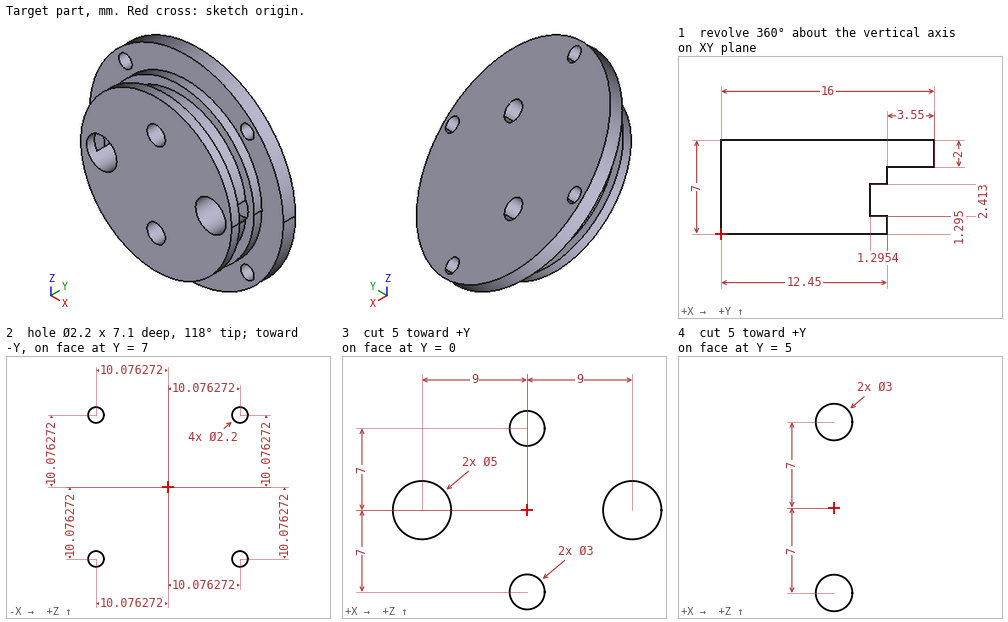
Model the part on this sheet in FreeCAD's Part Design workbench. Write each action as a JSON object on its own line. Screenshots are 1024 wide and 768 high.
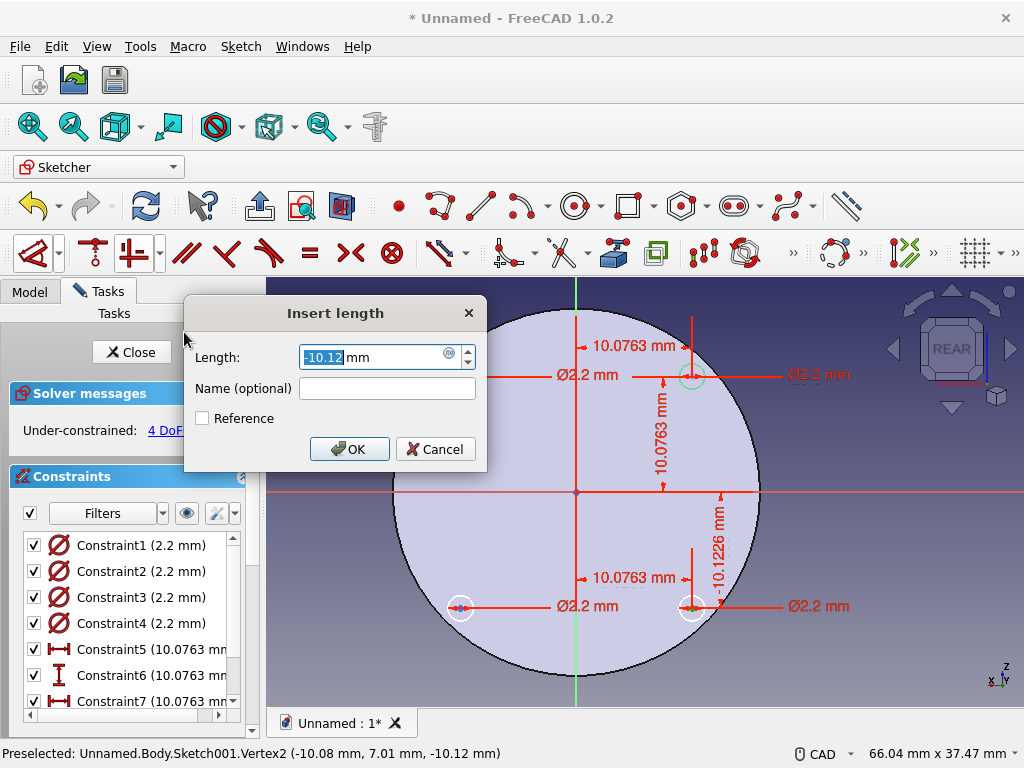
{"action": "type", "text": "-10.076272"}
{"action": "key", "text": "Return"}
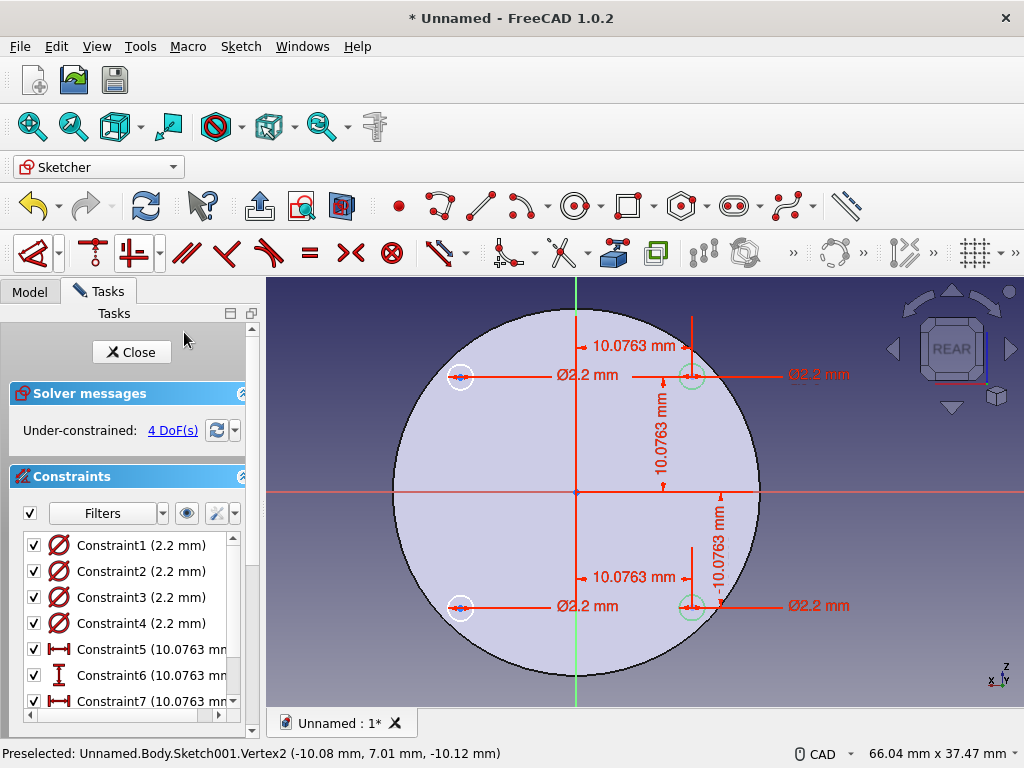
{"action": "left_click", "coordinate": [461, 608]}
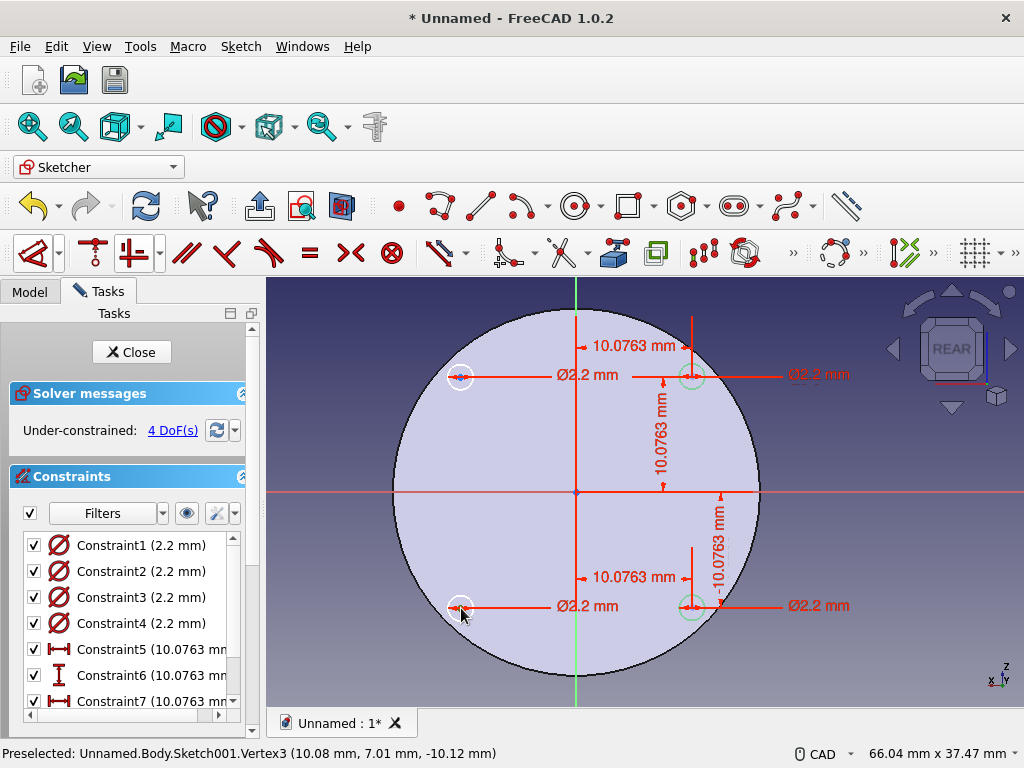
{"action": "left_click", "coordinate": [58, 254]}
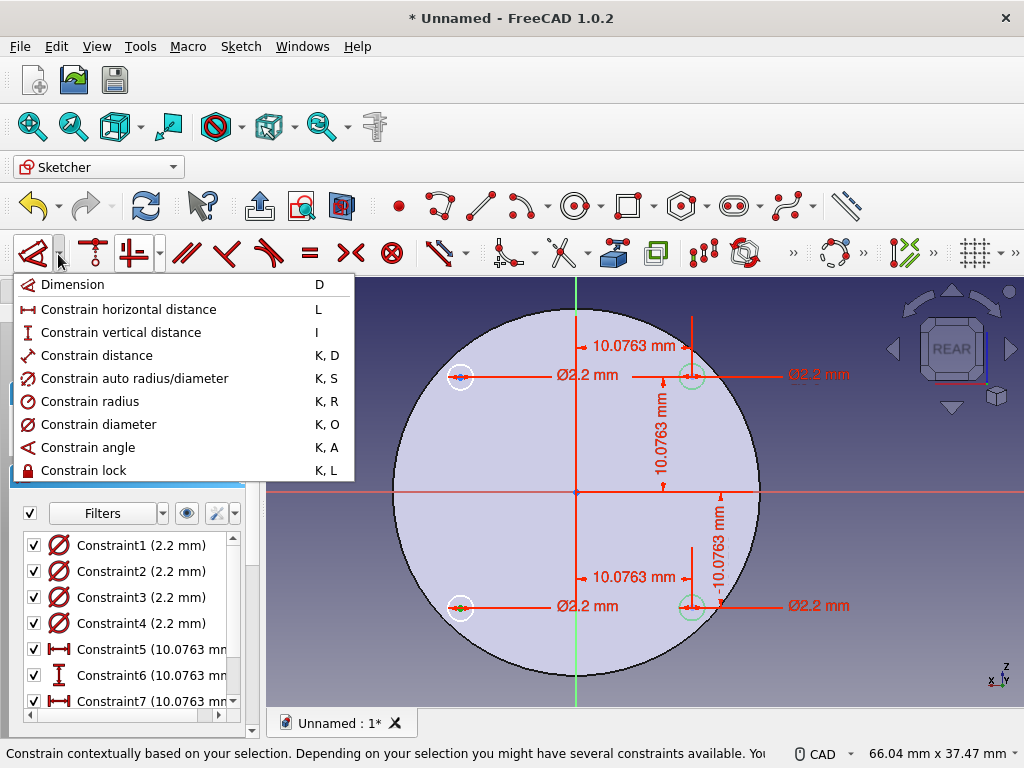
{"action": "left_click", "coordinate": [184, 310]}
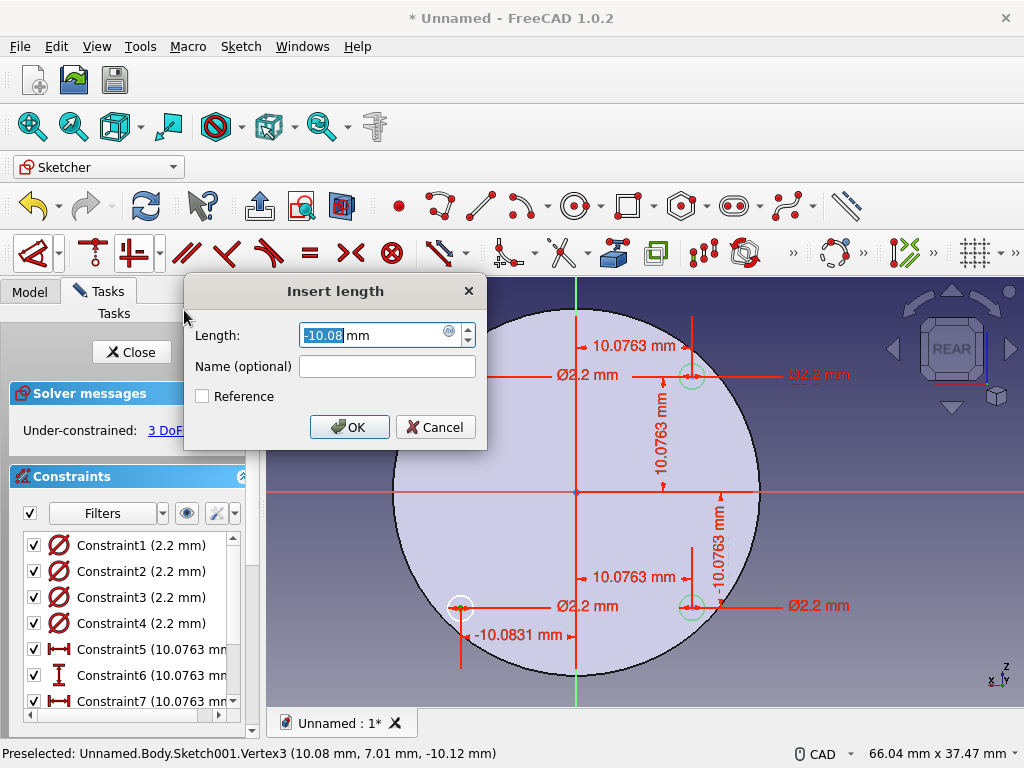
{"action": "type", "text": "-10.076272"}
{"action": "key", "text": "Return"}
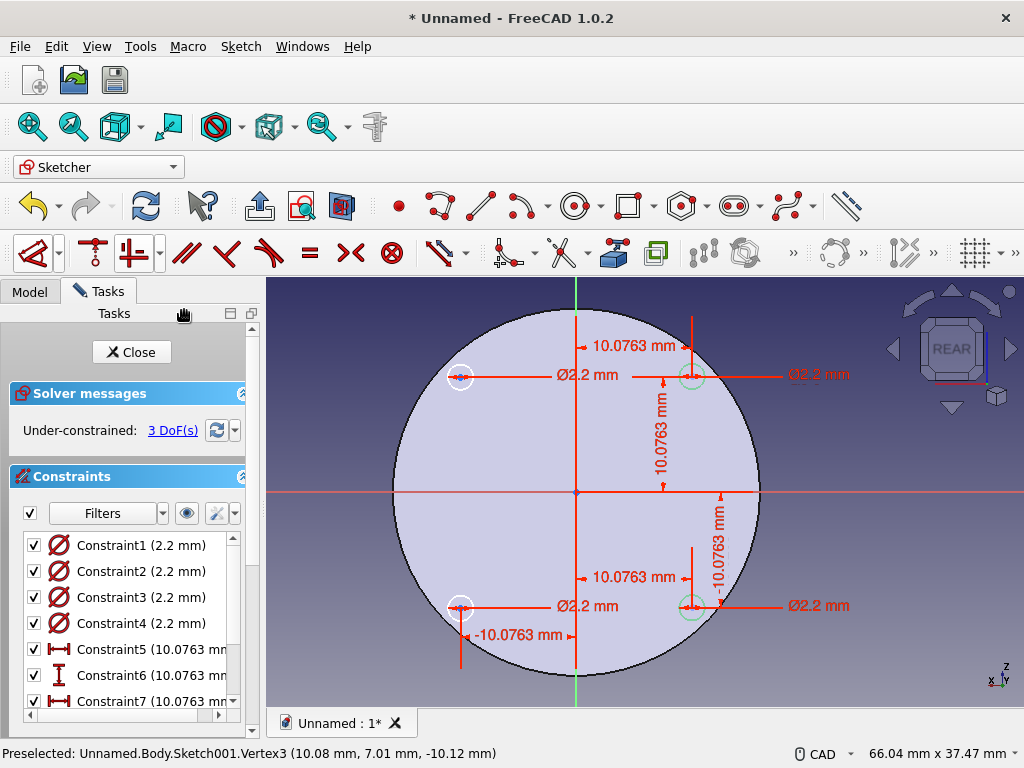
{"action": "left_click", "coordinate": [461, 608]}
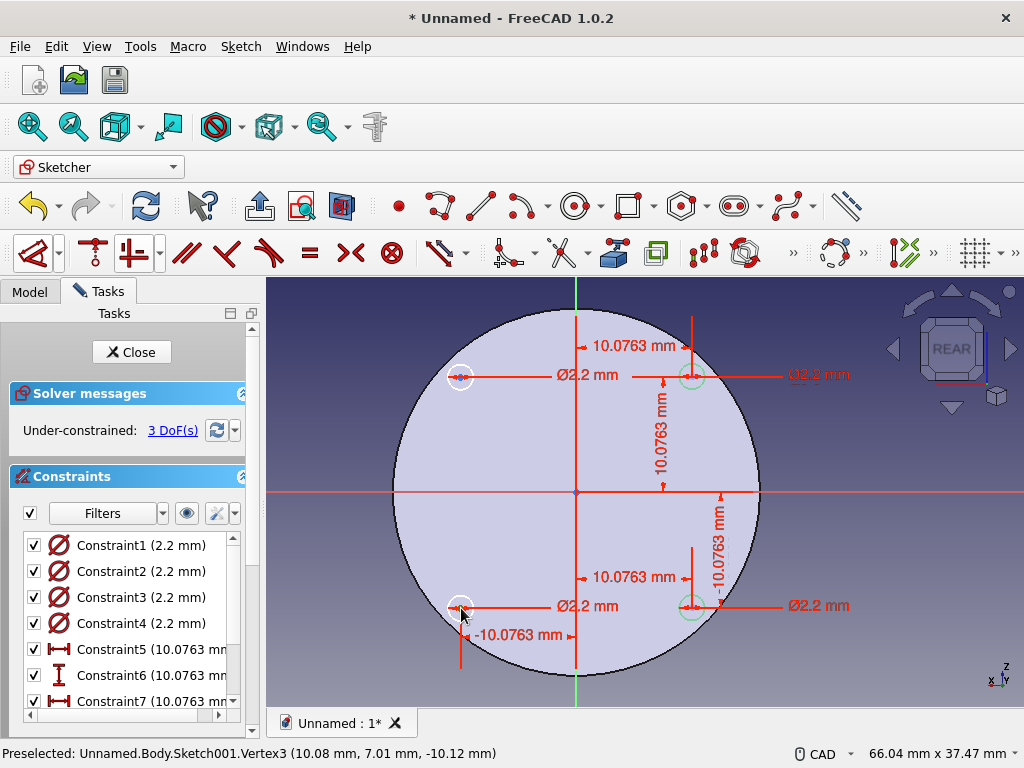
{"action": "left_click", "coordinate": [58, 254]}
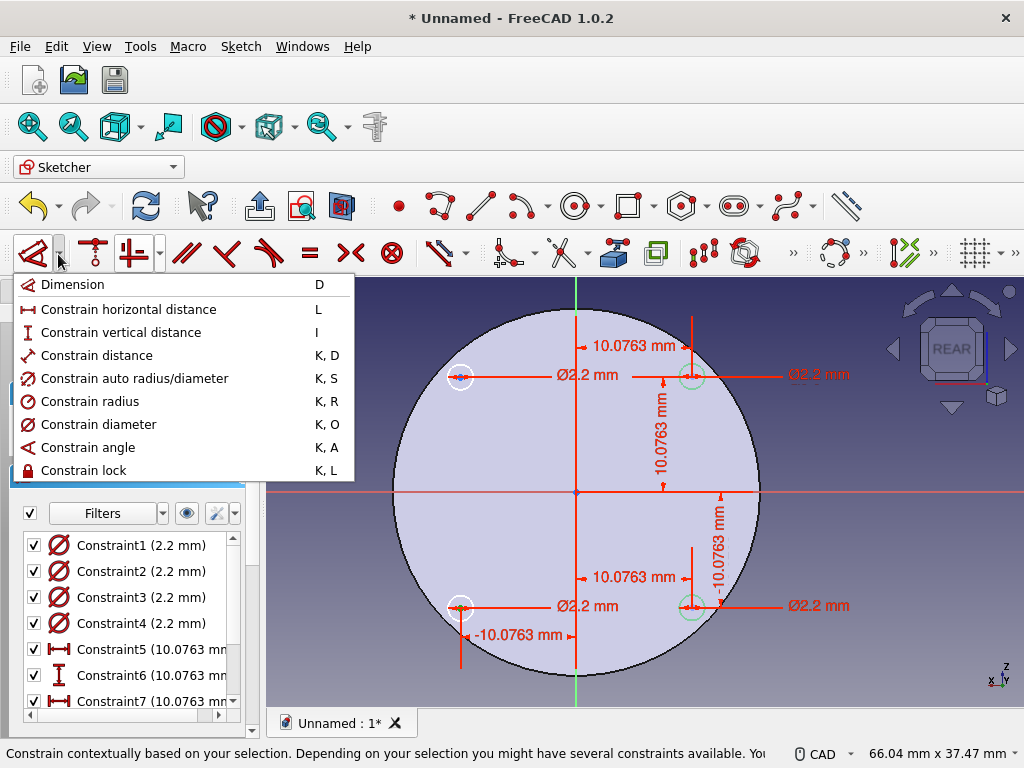
{"action": "left_click", "coordinate": [184, 332]}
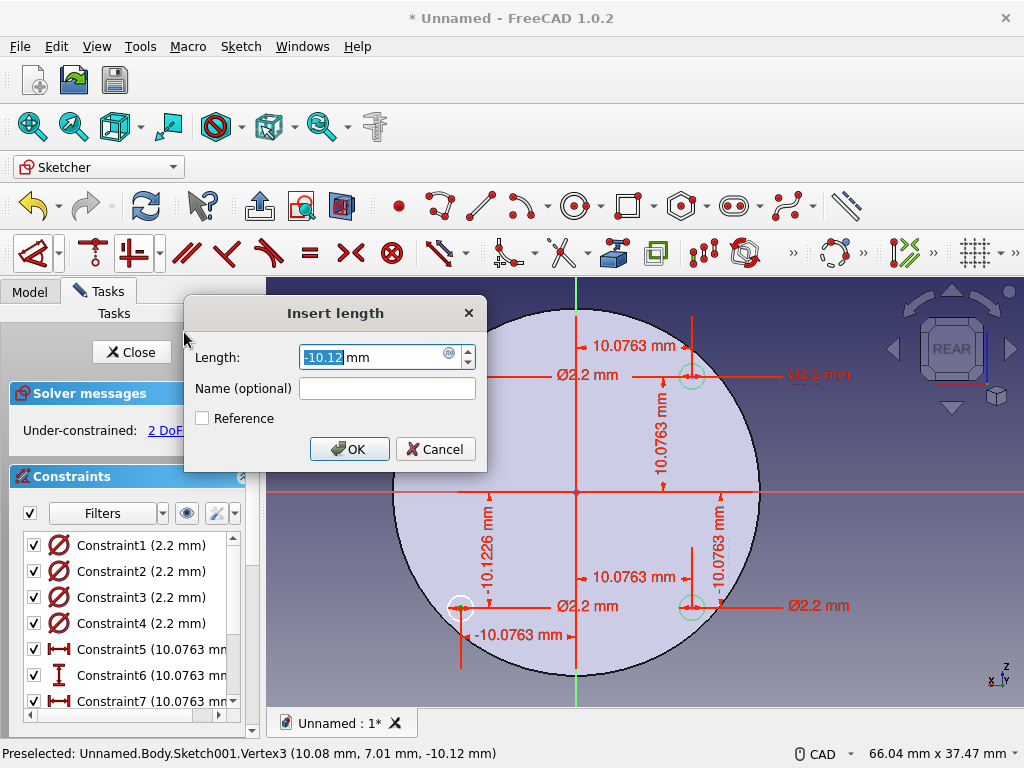
{"action": "type", "text": "-10.076272"}
{"action": "key", "text": "Return"}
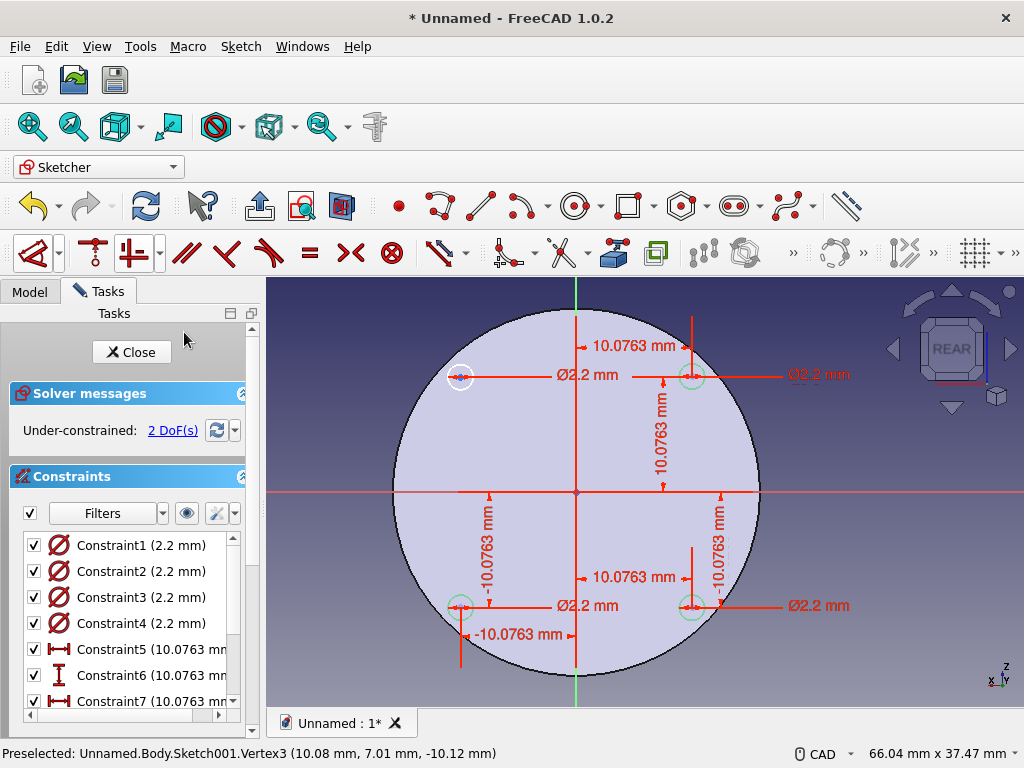
{"action": "left_click", "coordinate": [461, 377]}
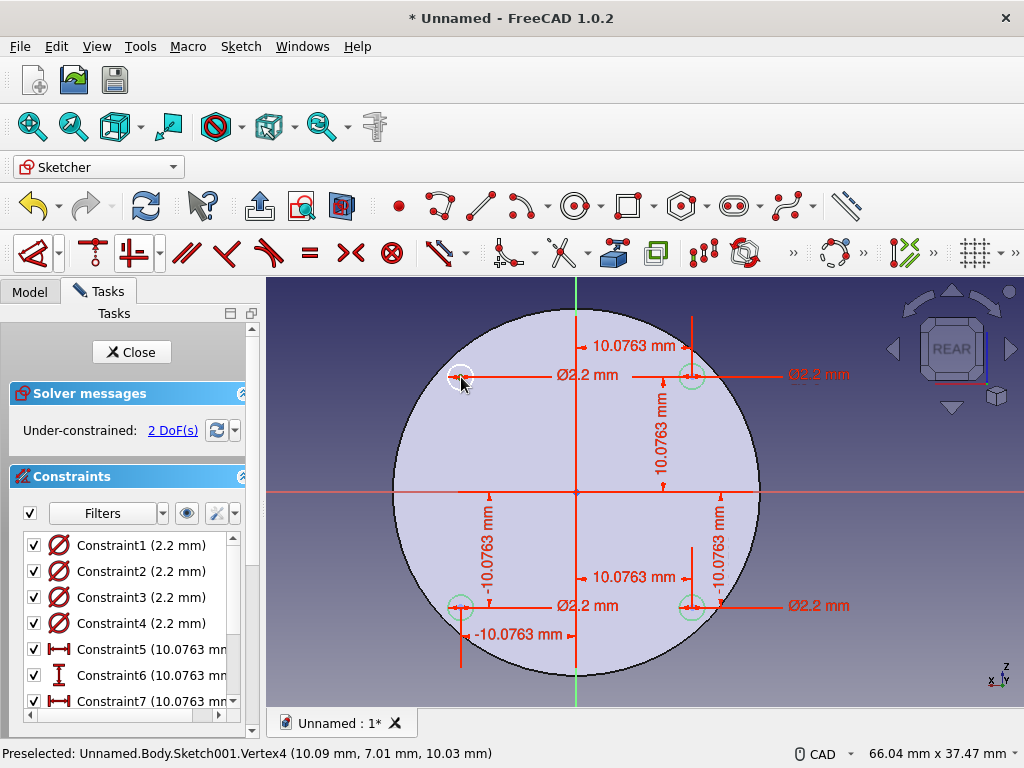
{"action": "key", "text": "l"}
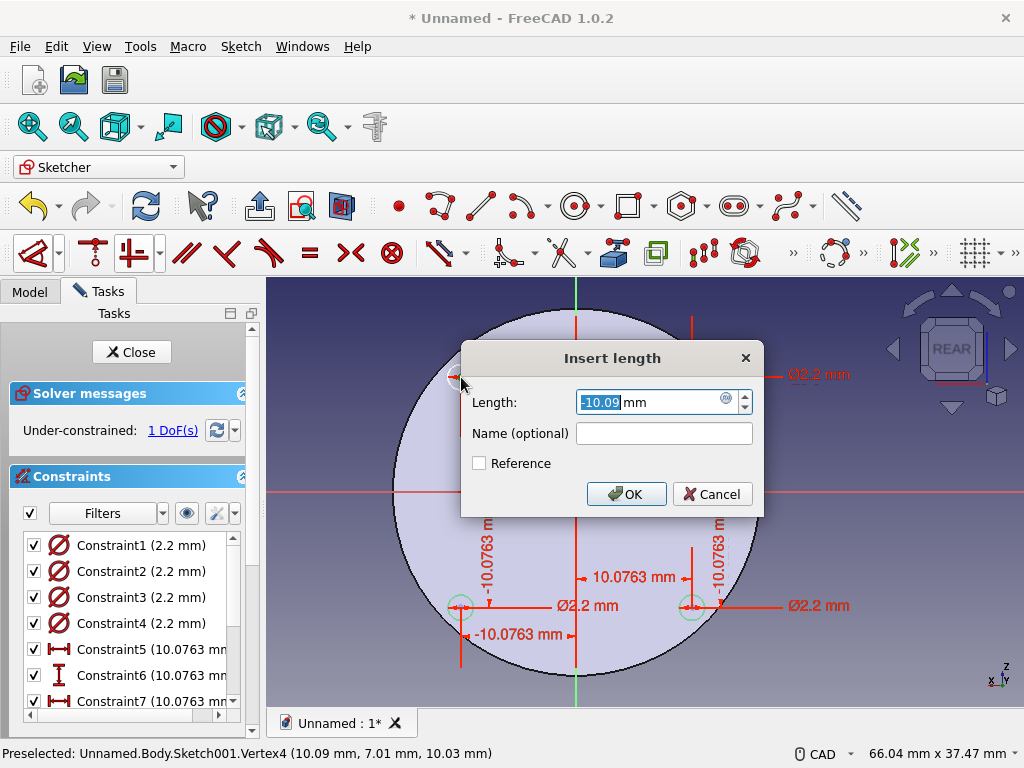
{"action": "type", "text": "-10.076272"}
{"action": "key", "text": "Return"}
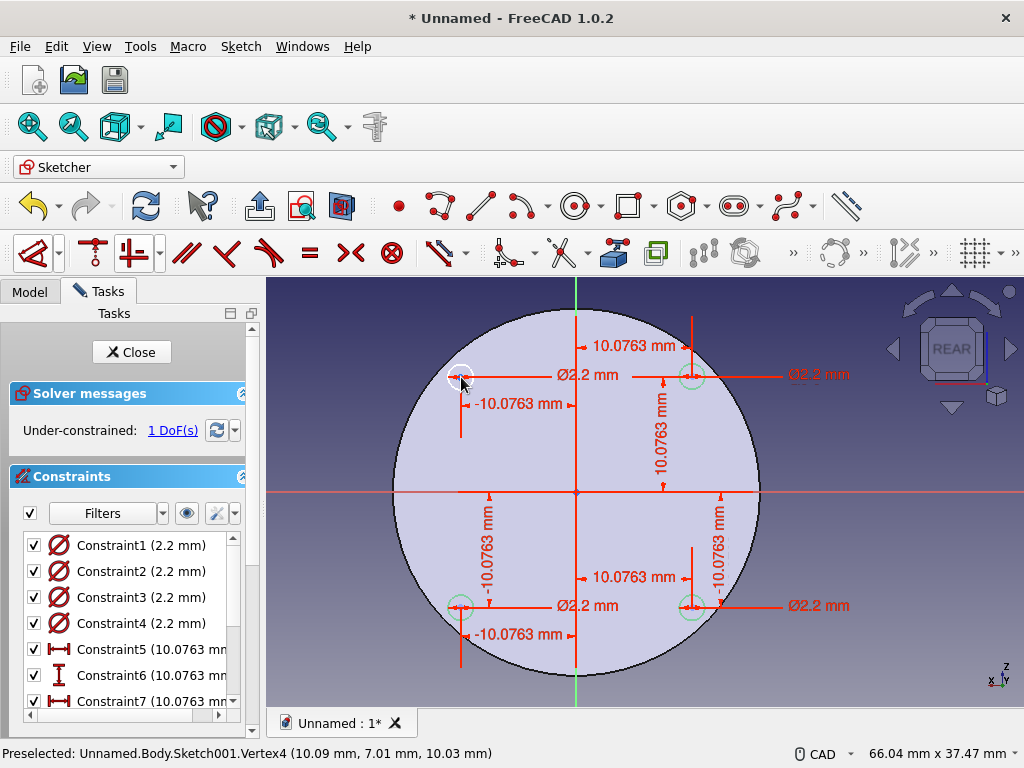
{"action": "left_click", "coordinate": [461, 377]}